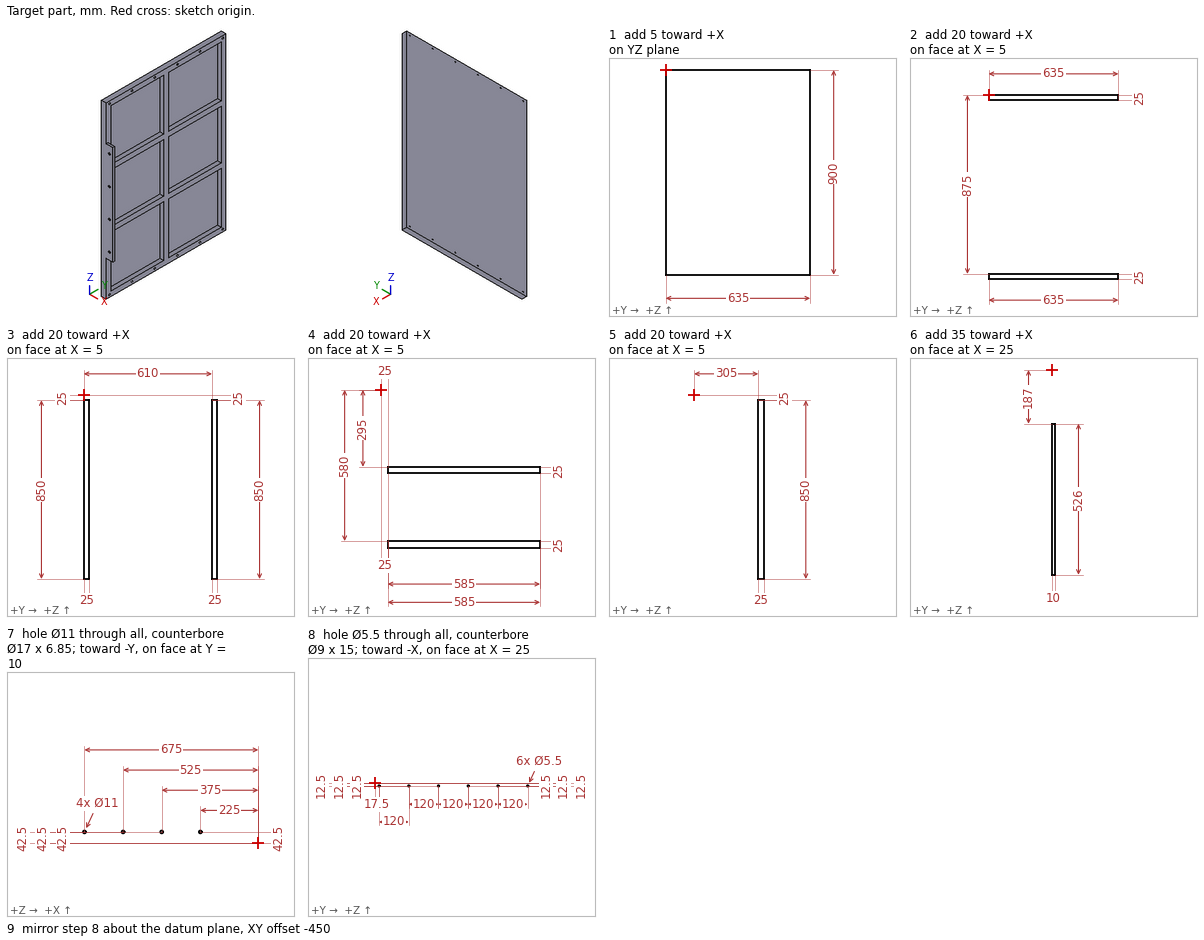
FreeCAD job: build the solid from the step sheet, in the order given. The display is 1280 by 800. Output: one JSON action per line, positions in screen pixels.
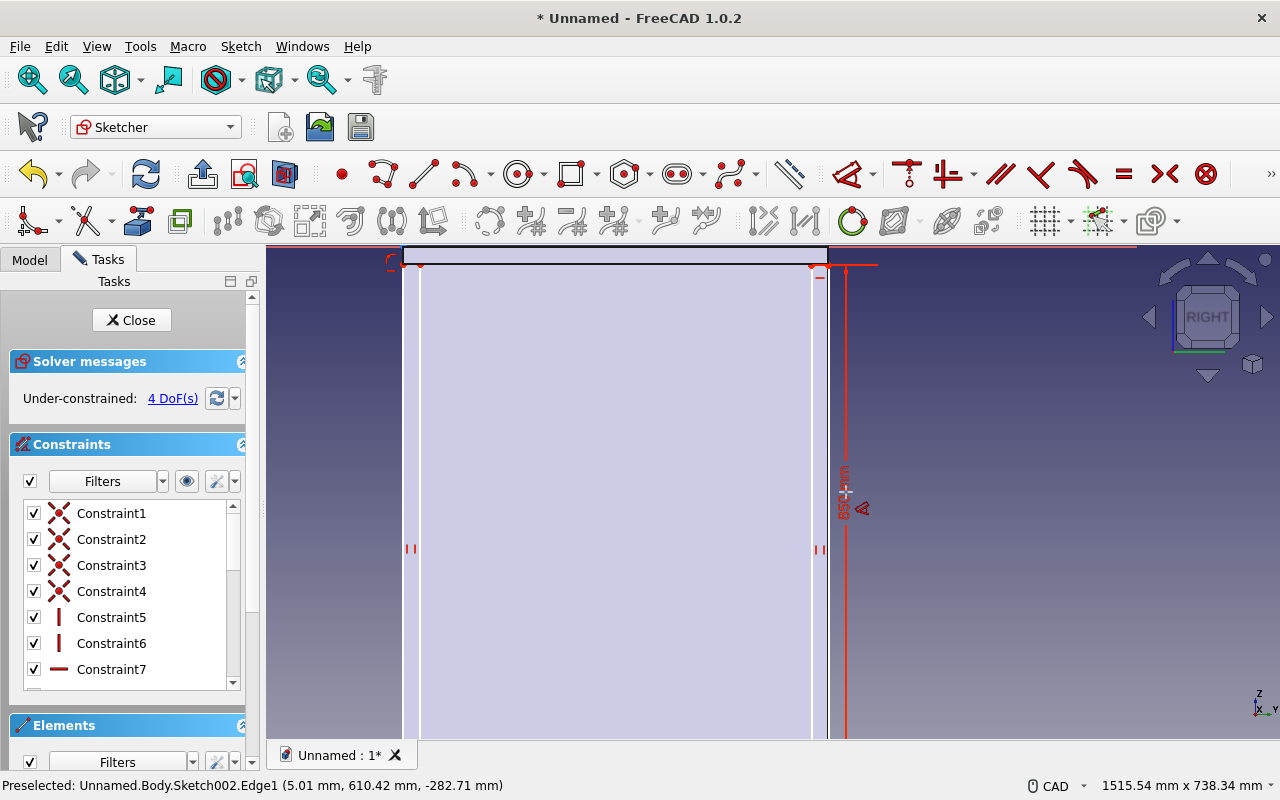
{"action": "left_click", "coordinate": [403, 435]}
{"action": "left_click", "coordinate": [369, 492]}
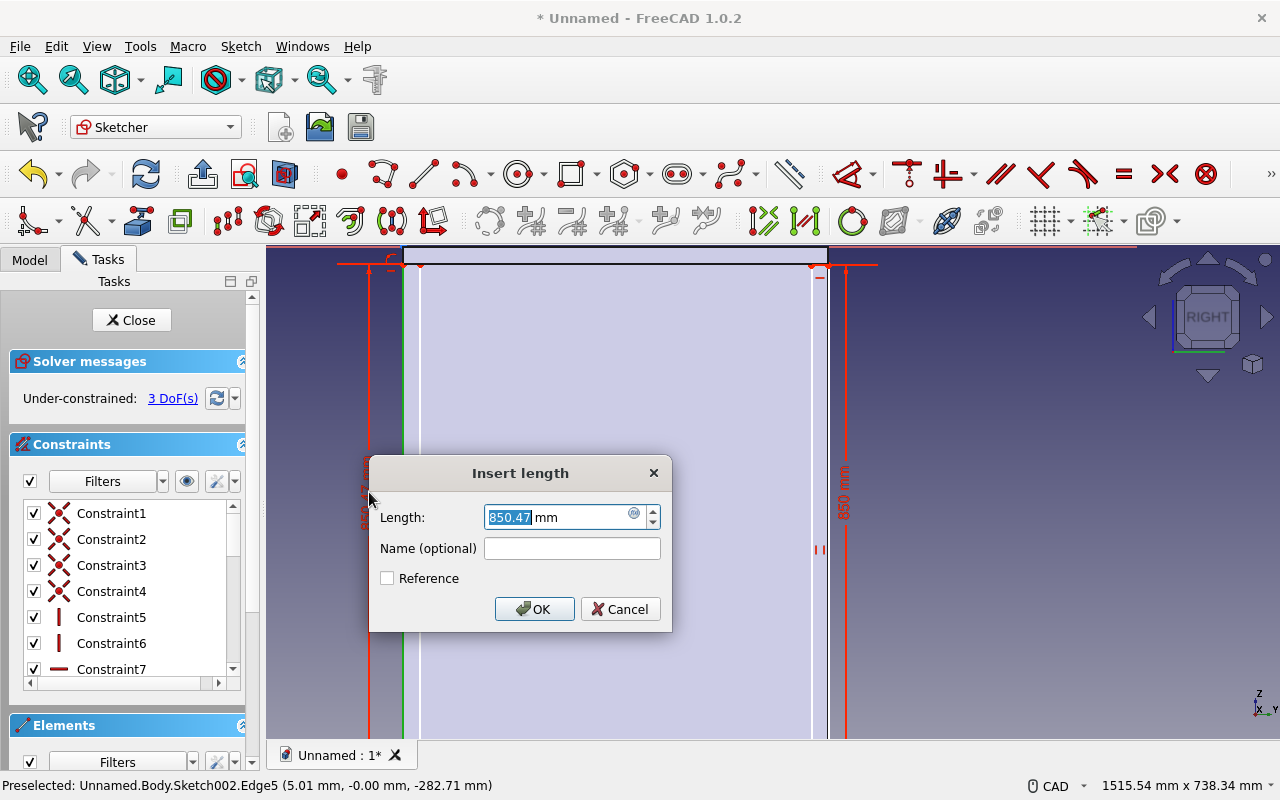
{"action": "type", "text": "850"}
{"action": "key", "text": "Return"}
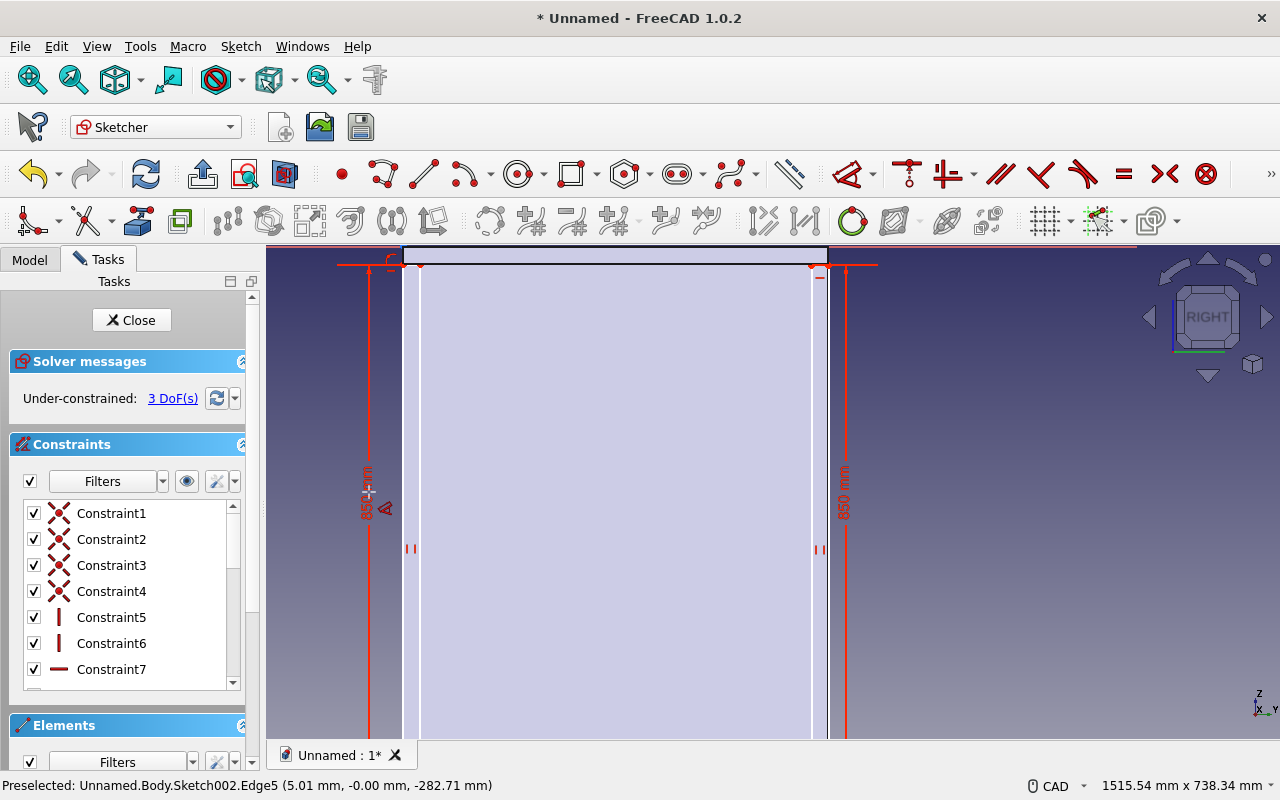
{"action": "scroll", "coordinate": [812, 434], "scroll_direction": "down", "scroll_amount": 3}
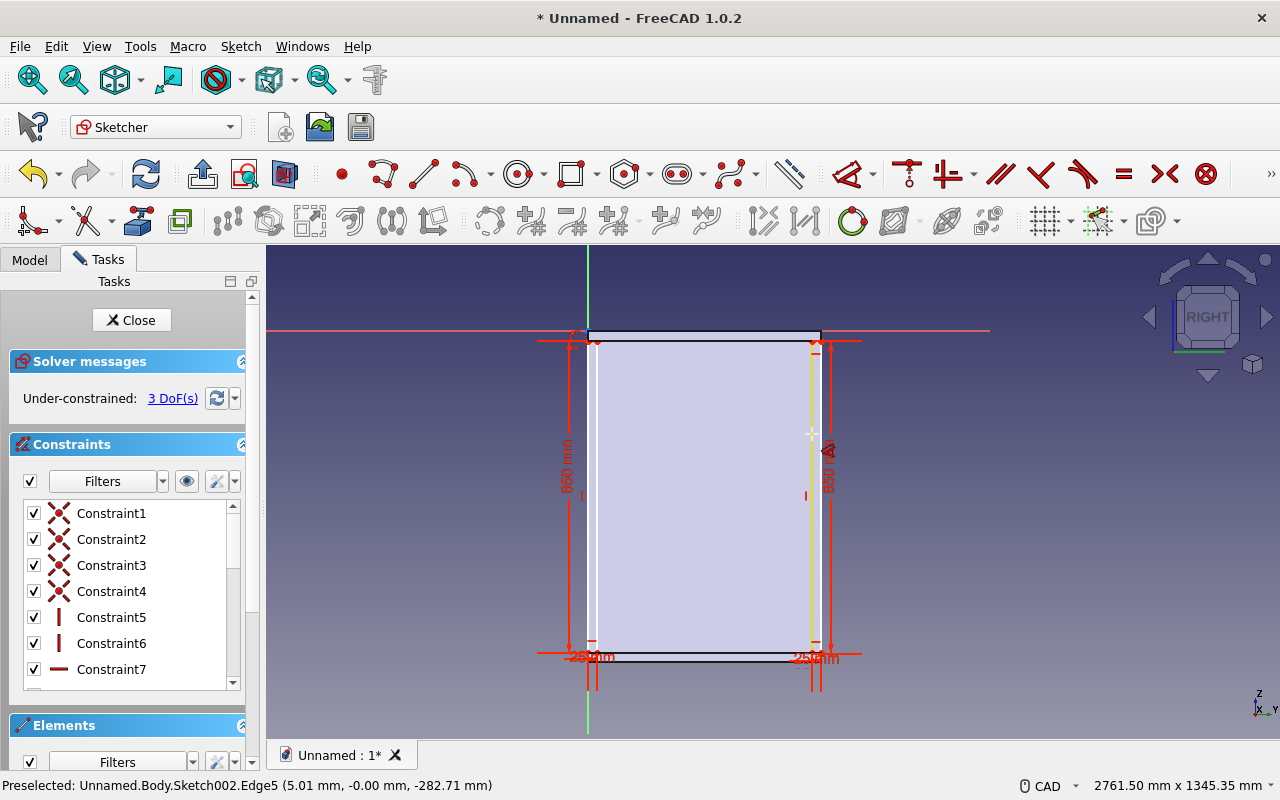
{"action": "scroll", "coordinate": [812, 341], "scroll_direction": "up", "scroll_amount": 8}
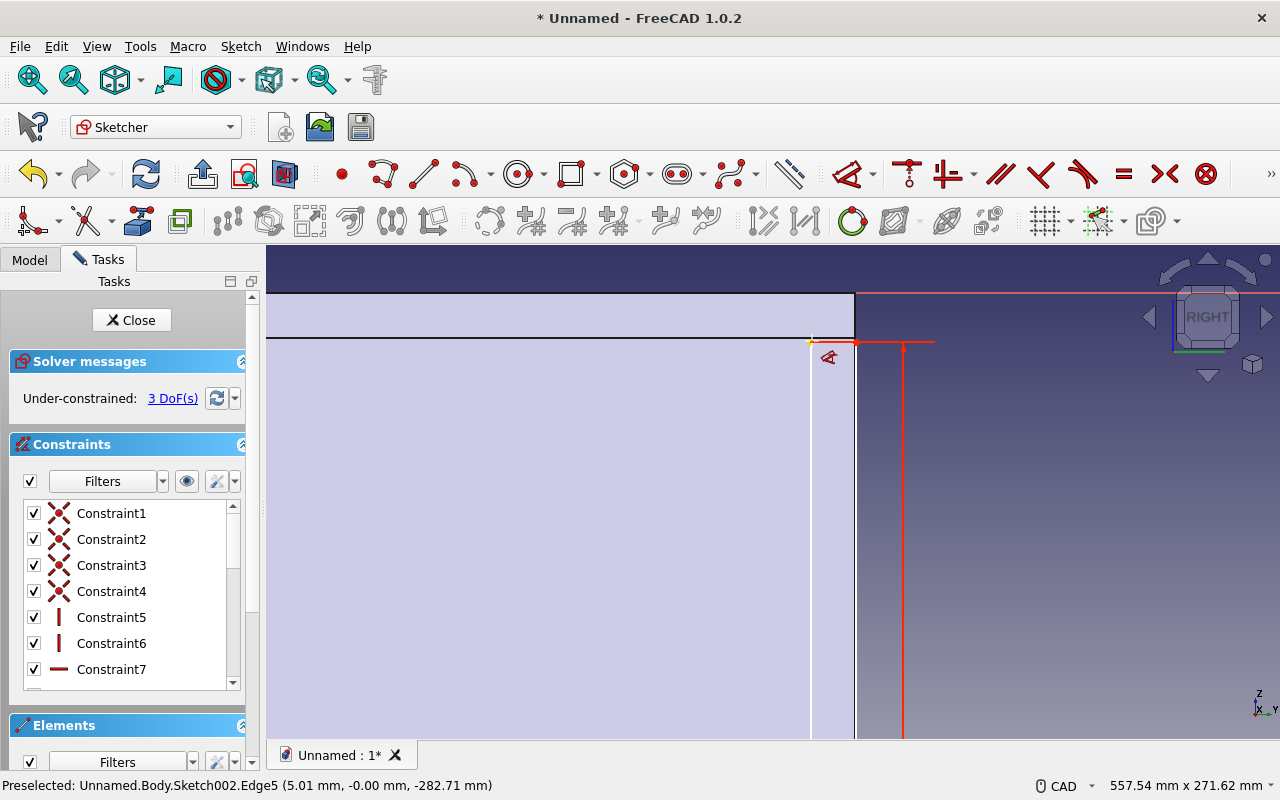
{"action": "left_click", "coordinate": [811, 342]}
{"action": "left_click", "coordinate": [845, 318]}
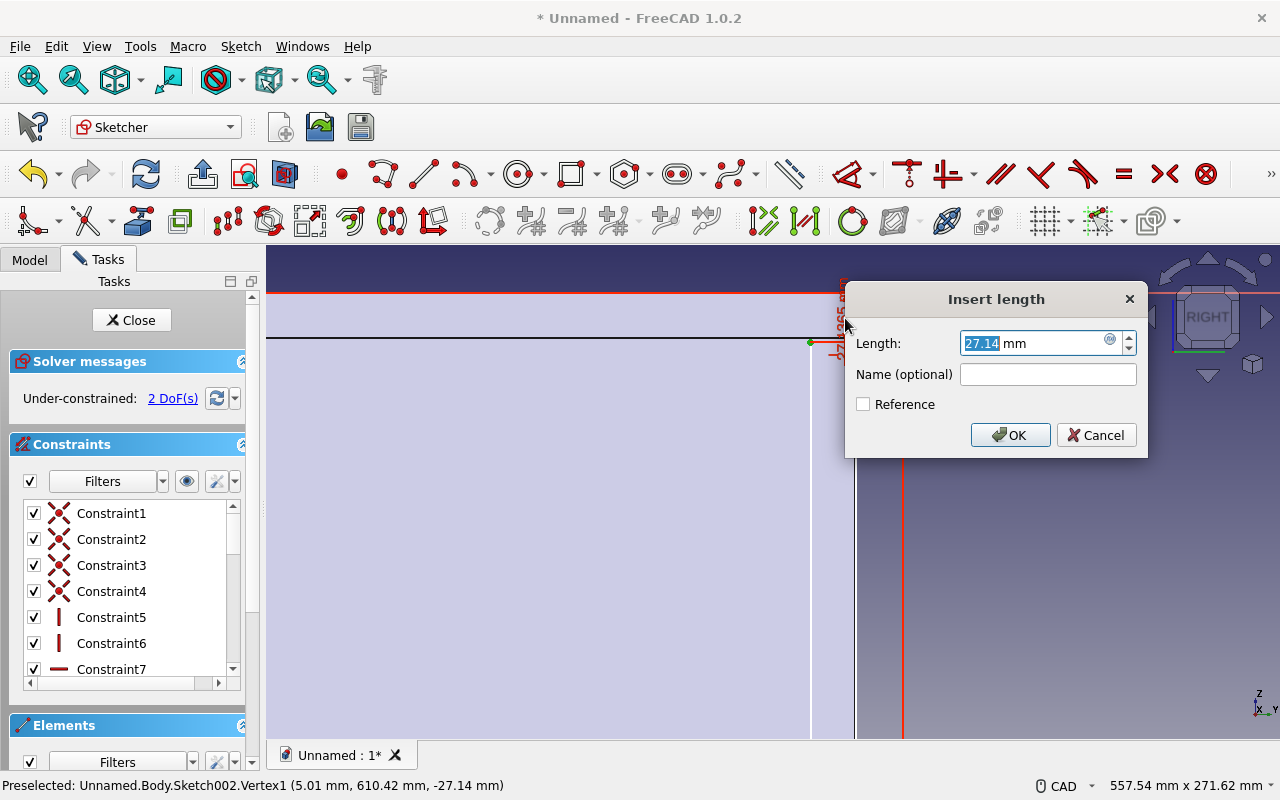
{"action": "type", "text": "25"}
{"action": "key", "text": "Return"}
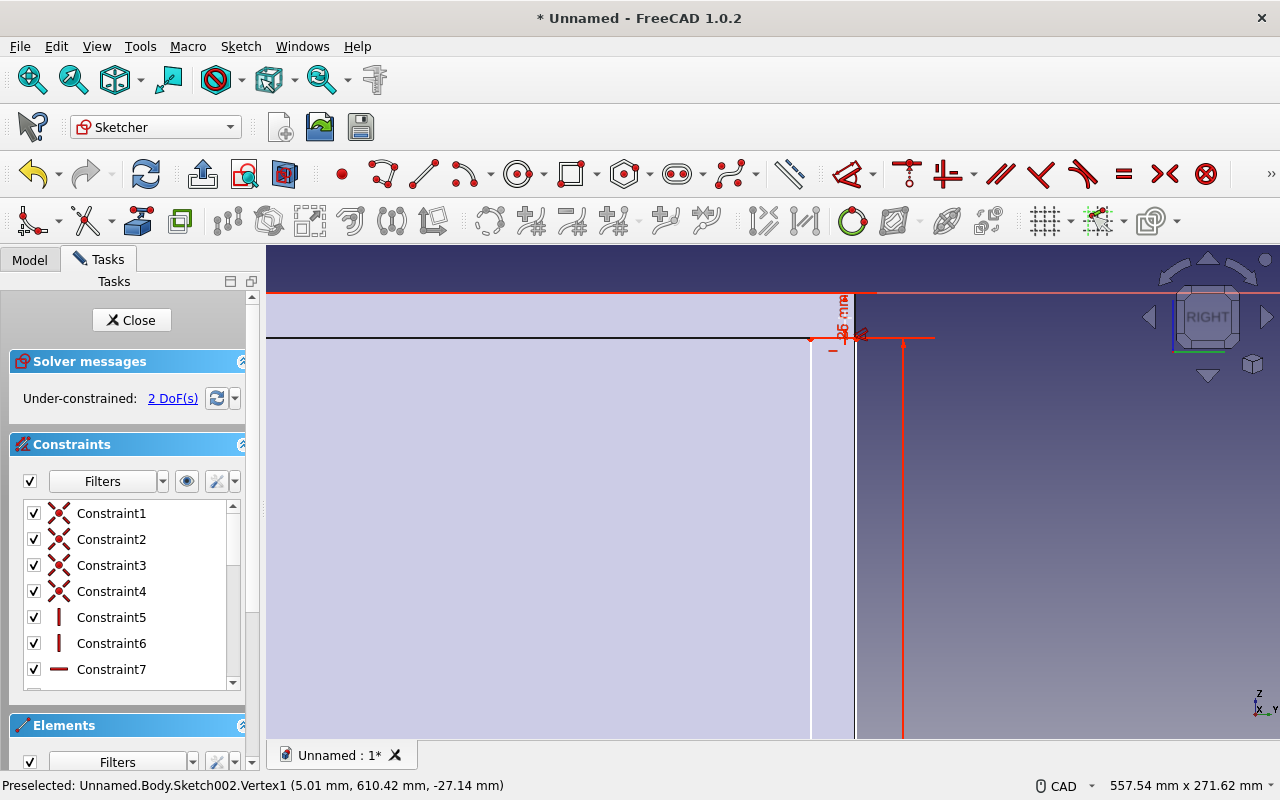
{"action": "scroll", "coordinate": [812, 341], "scroll_direction": "down", "scroll_amount": 8}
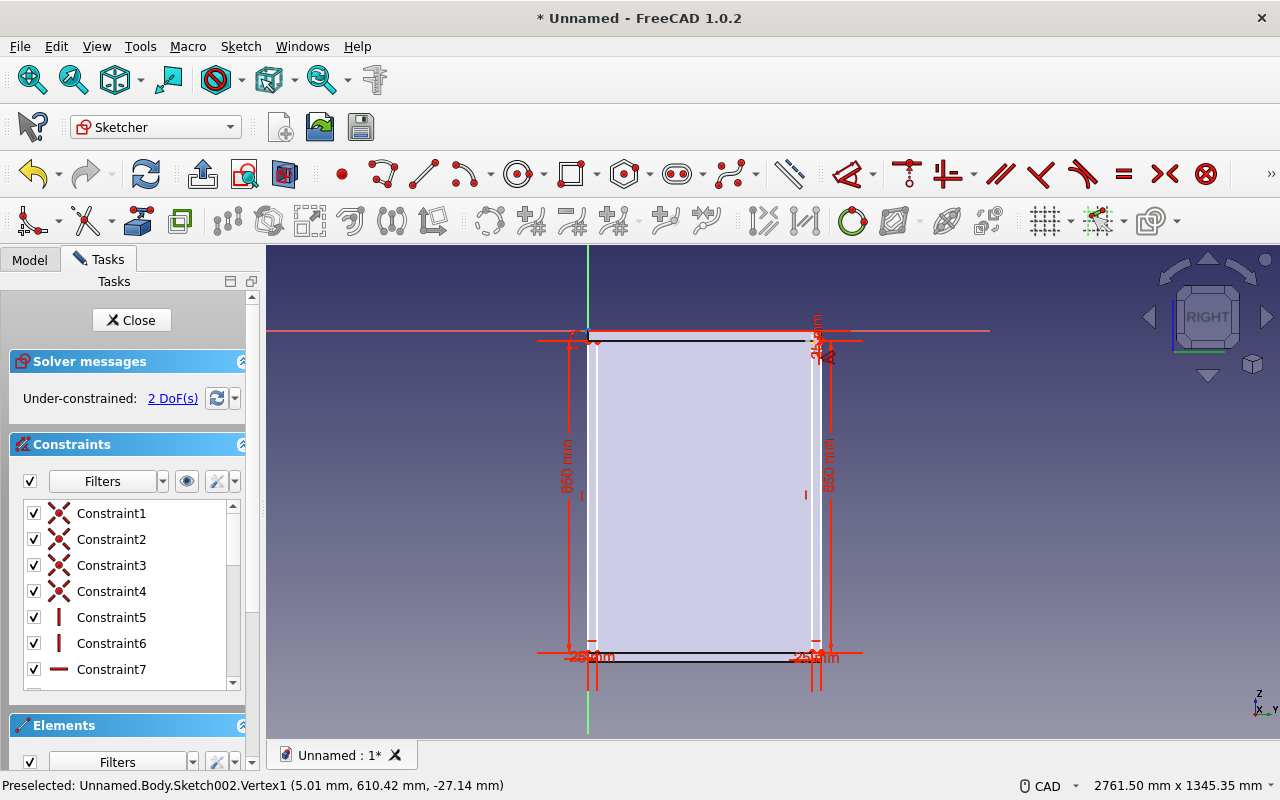
{"action": "scroll", "coordinate": [588, 341], "scroll_direction": "up", "scroll_amount": 8}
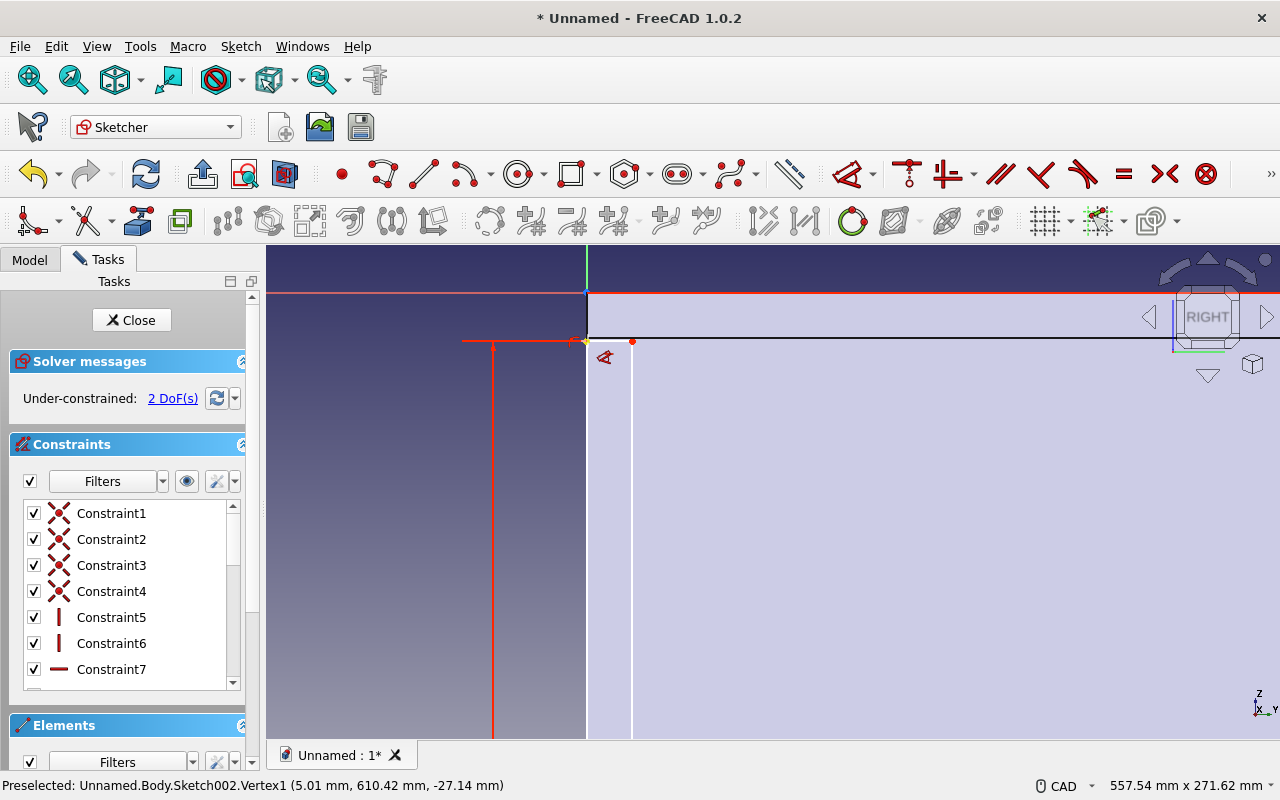
{"action": "left_click", "coordinate": [587, 341]}
{"action": "left_click", "coordinate": [553, 317]}